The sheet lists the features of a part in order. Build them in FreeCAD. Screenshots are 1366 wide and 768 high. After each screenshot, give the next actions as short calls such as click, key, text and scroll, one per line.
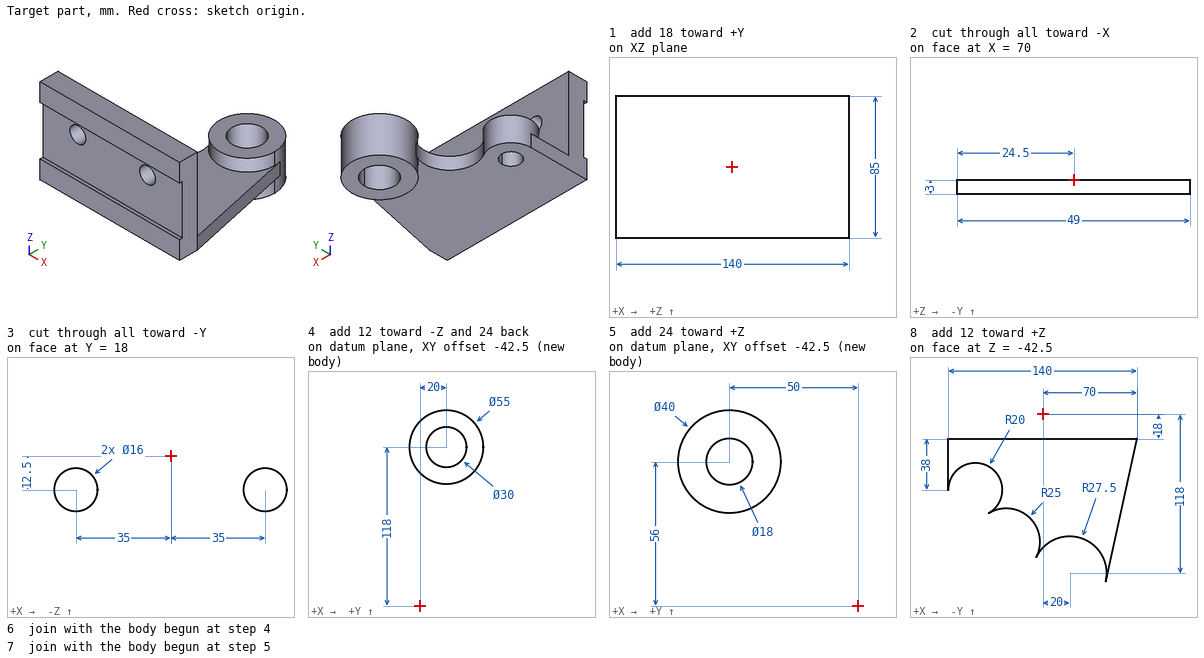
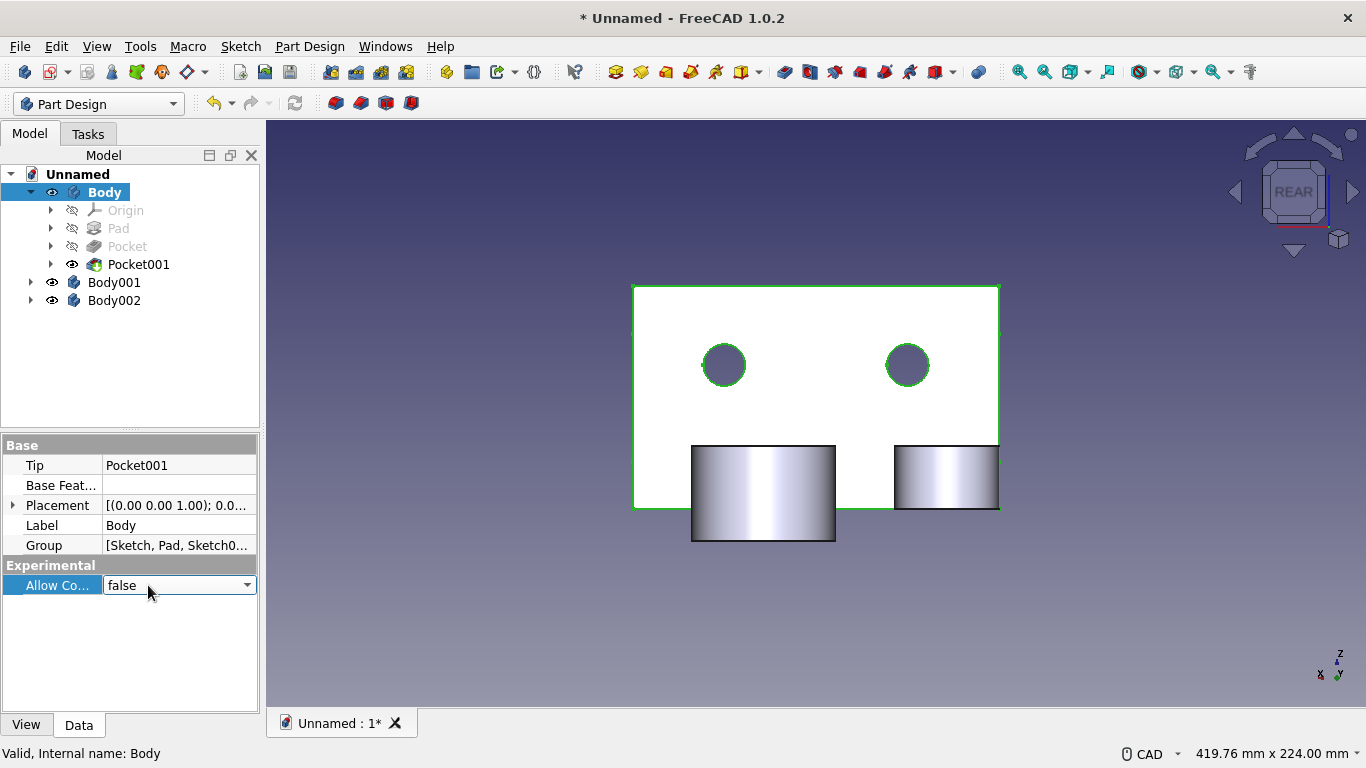
click(148, 585)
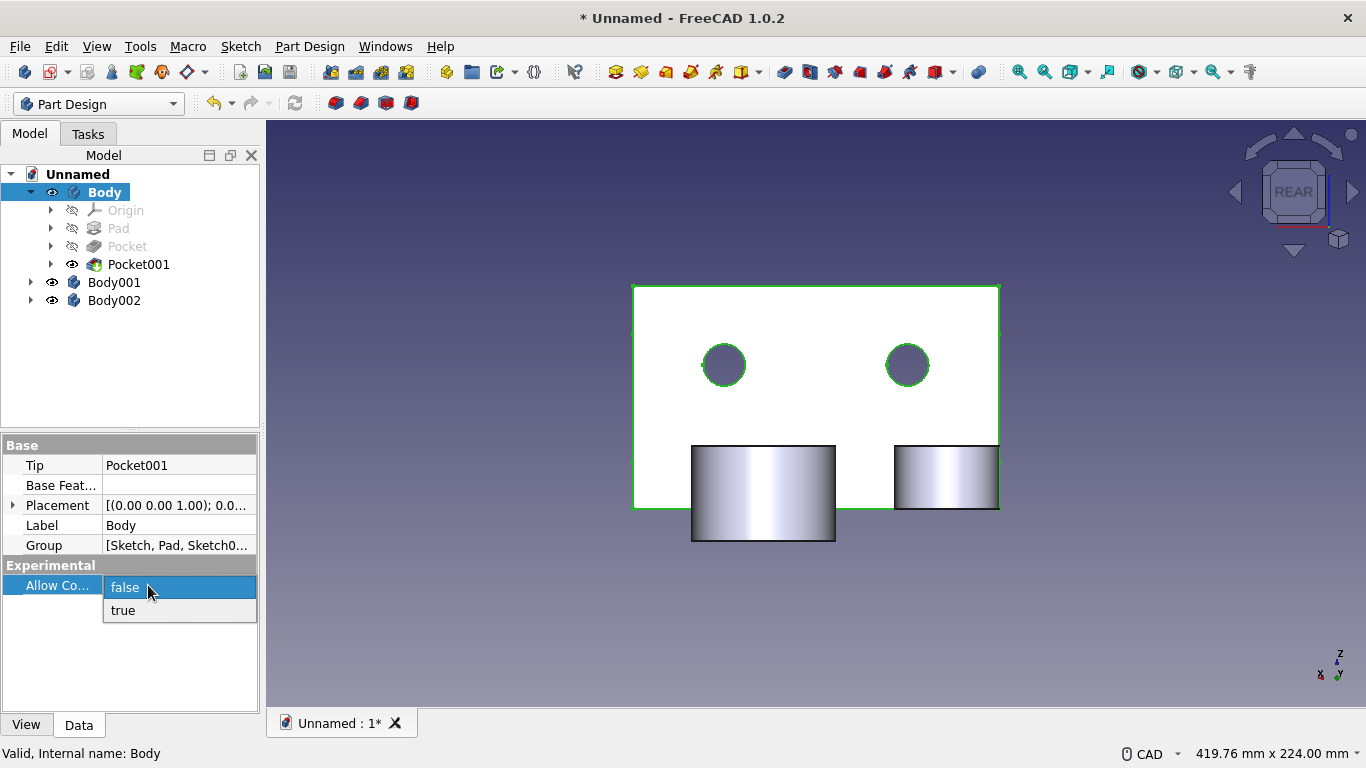
click(178, 610)
key(Return)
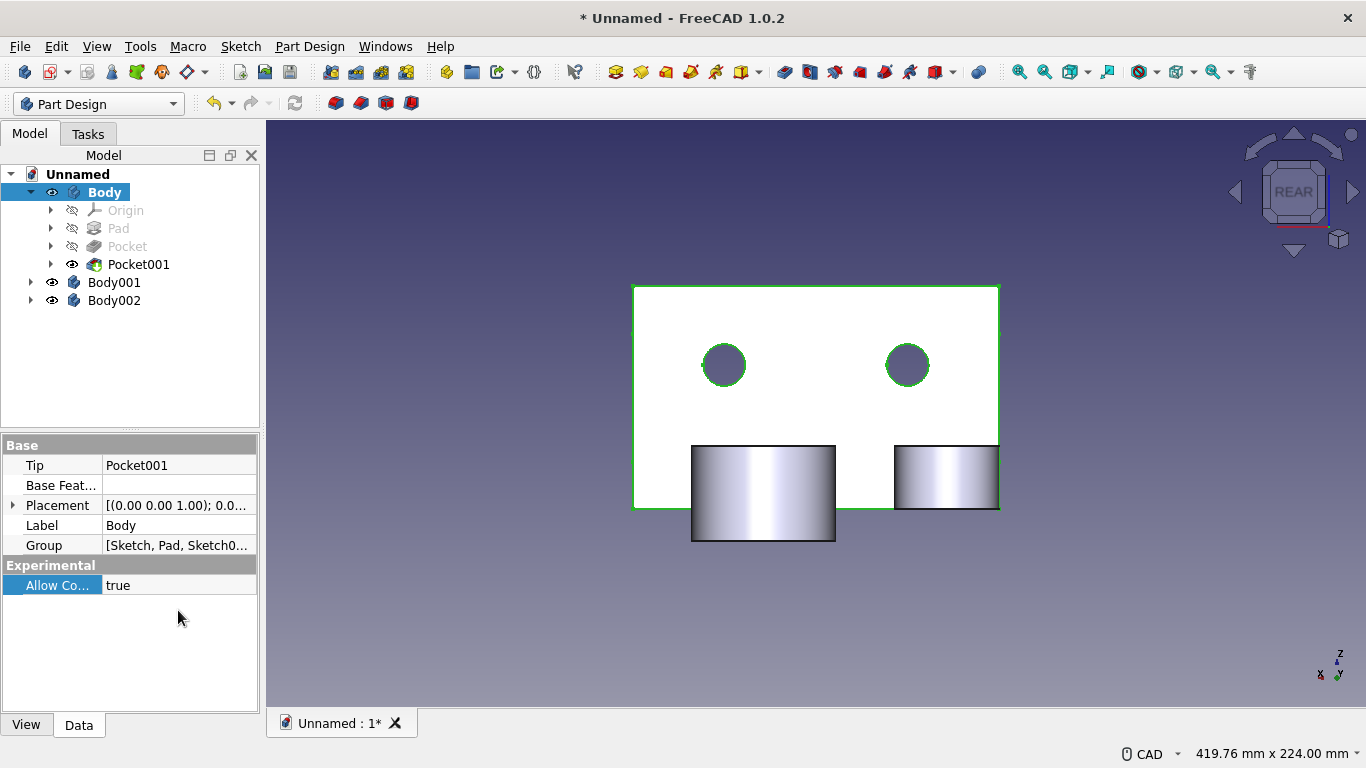
click(97, 282)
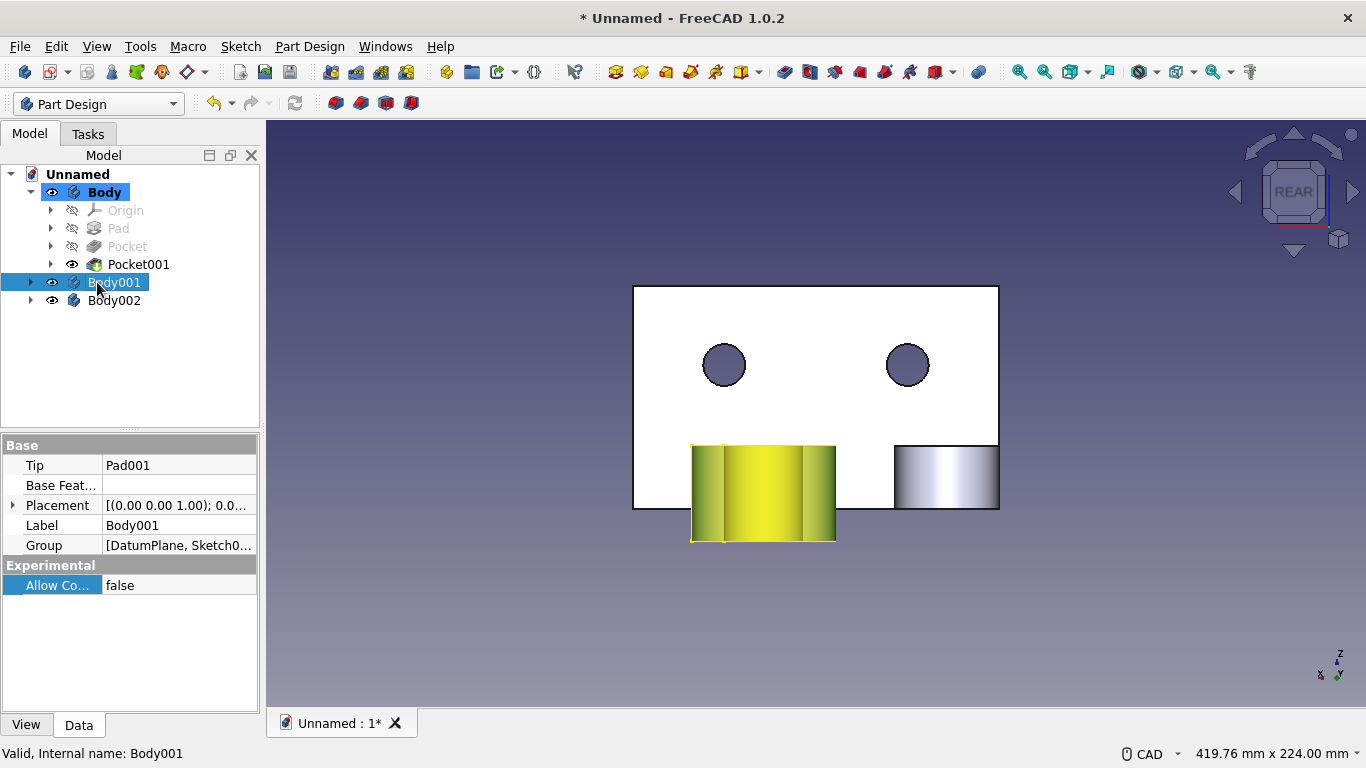
click(979, 72)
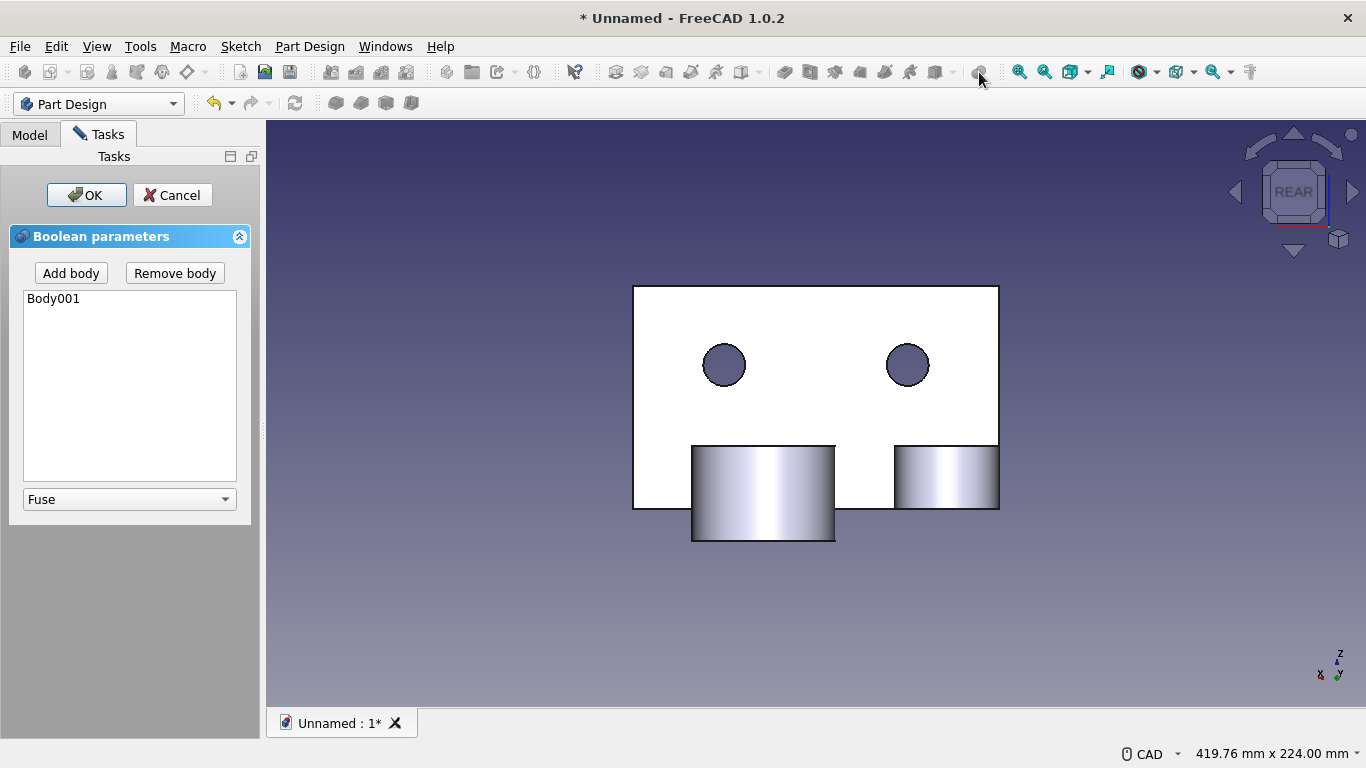
click(87, 195)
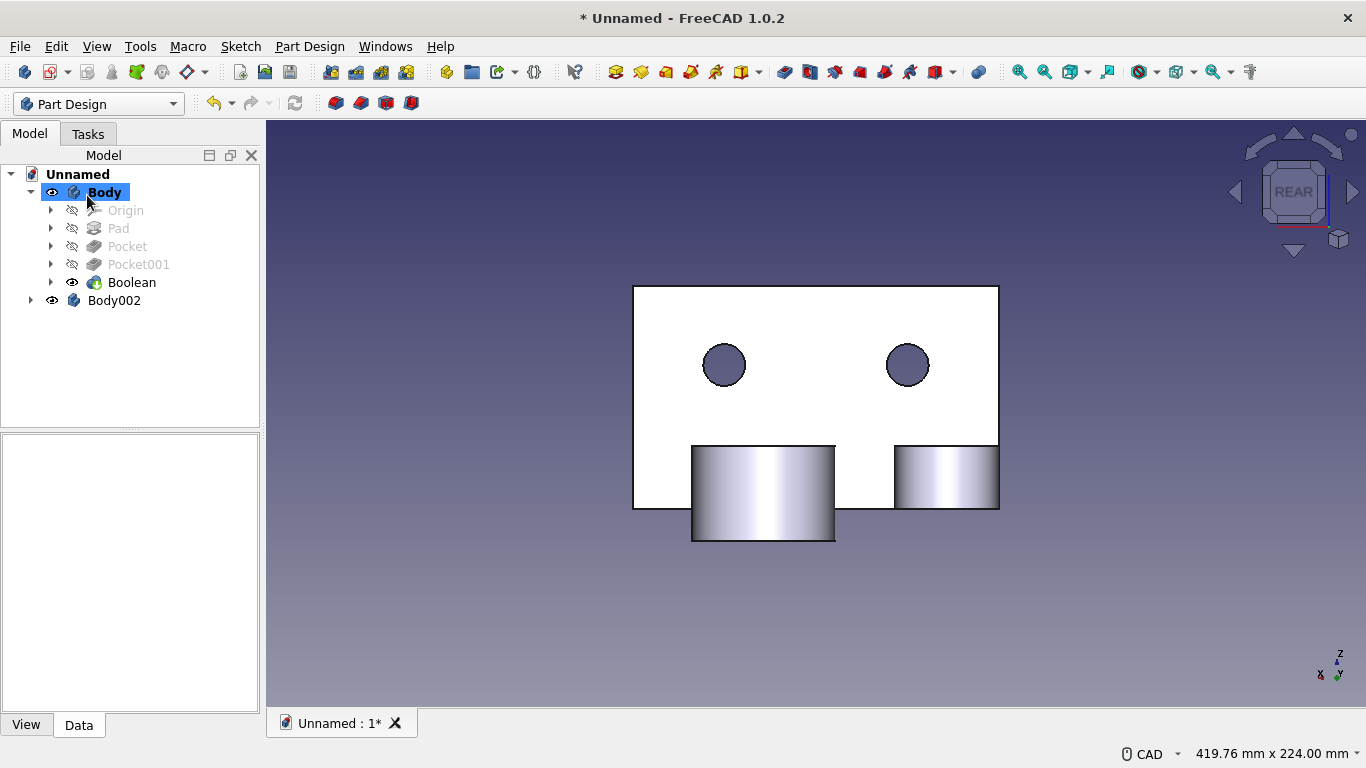
click(1020, 72)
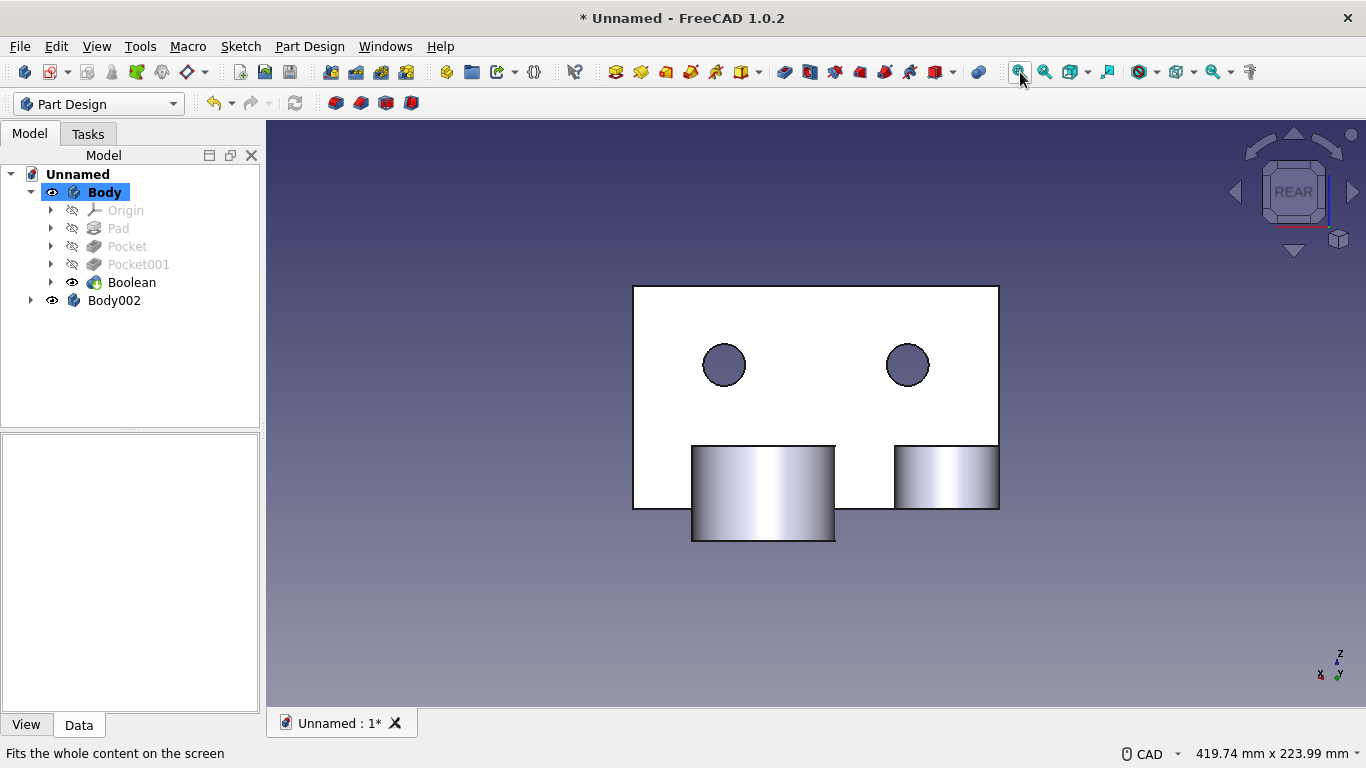
click(97, 300)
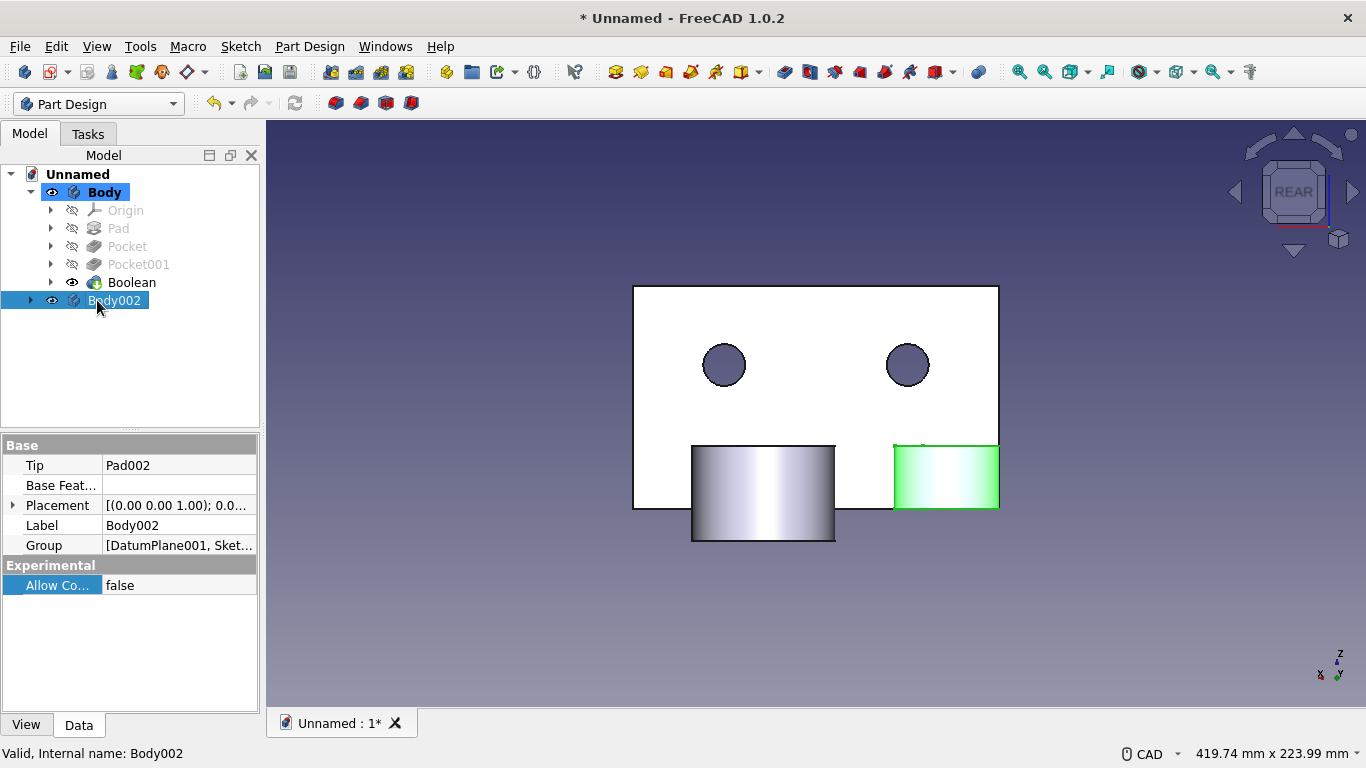
click(979, 72)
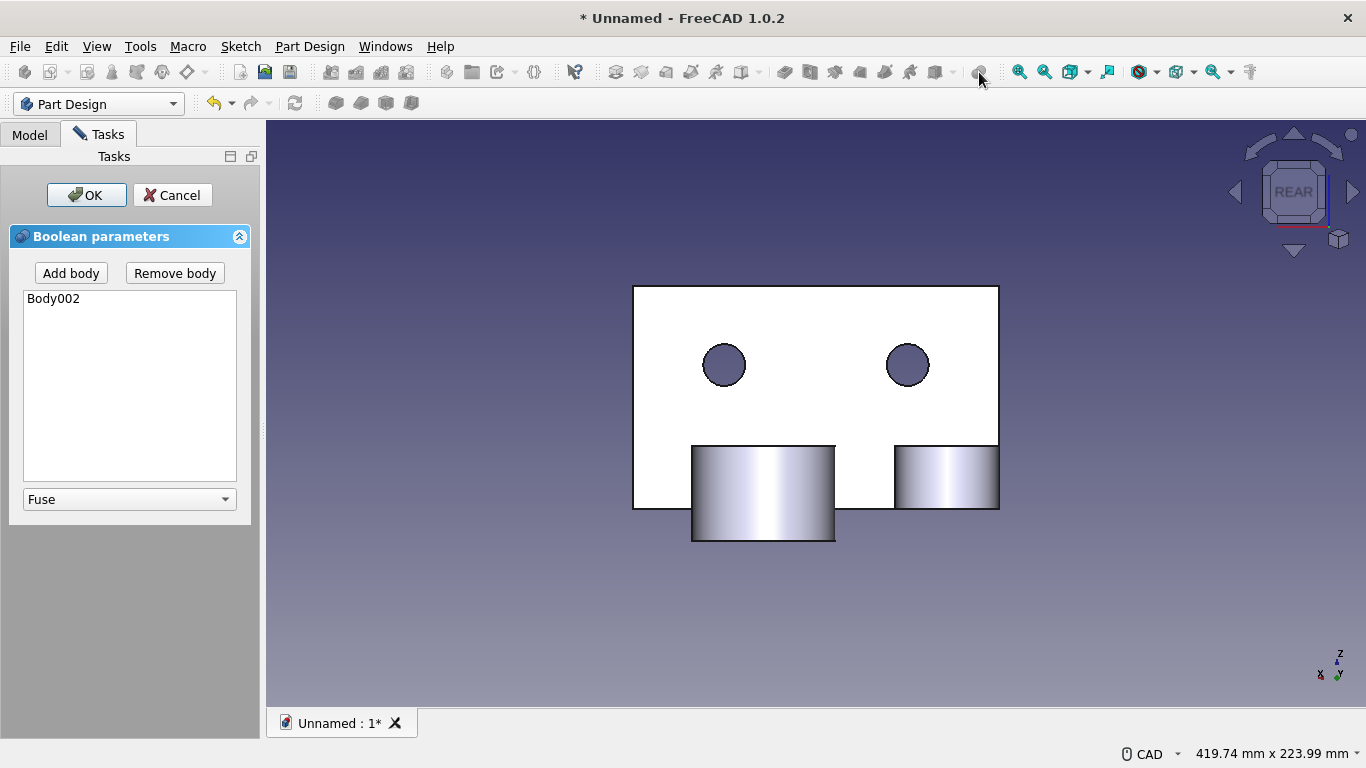
click(87, 195)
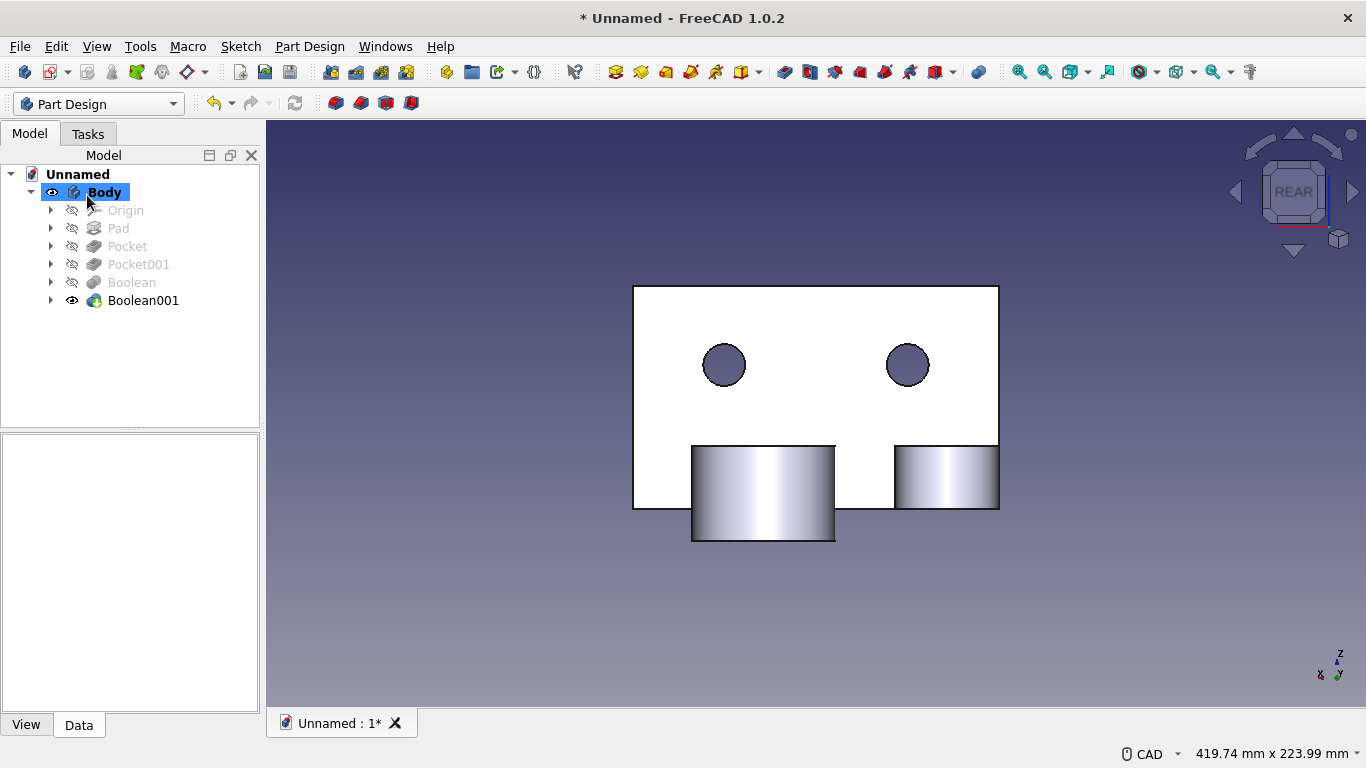
click(1020, 72)